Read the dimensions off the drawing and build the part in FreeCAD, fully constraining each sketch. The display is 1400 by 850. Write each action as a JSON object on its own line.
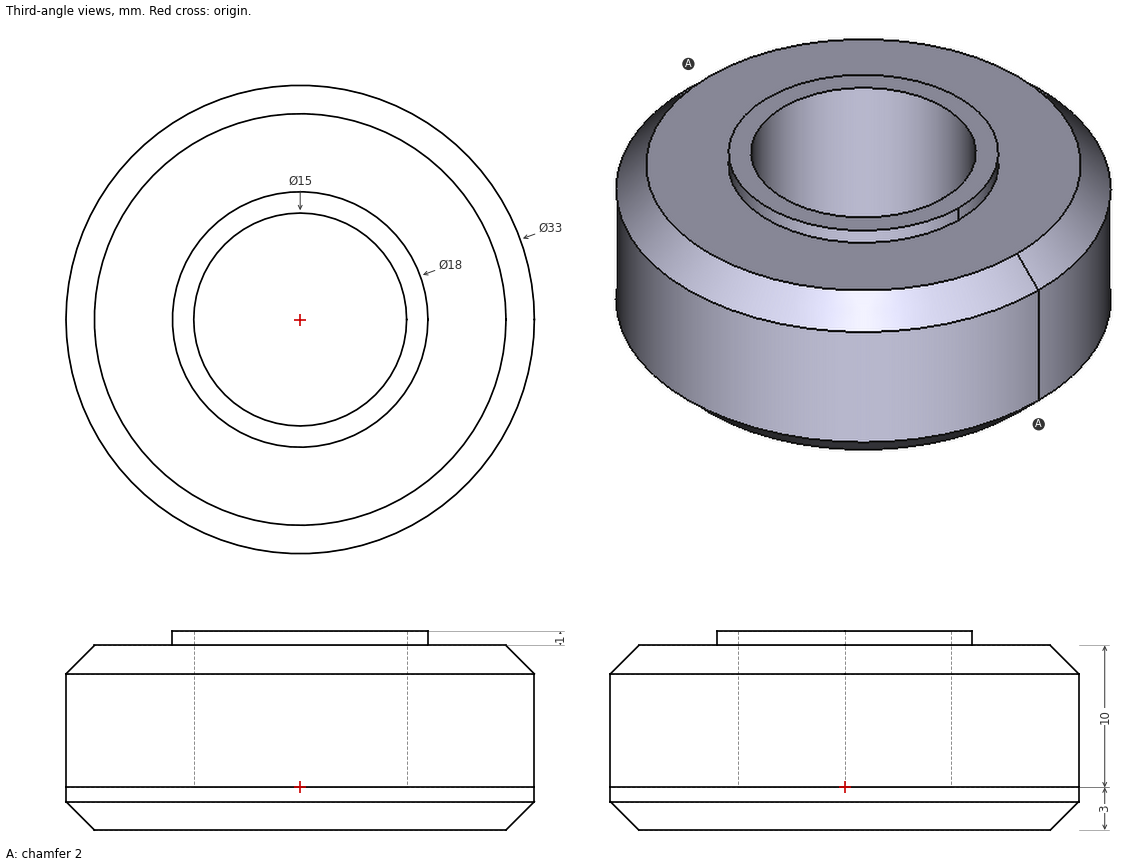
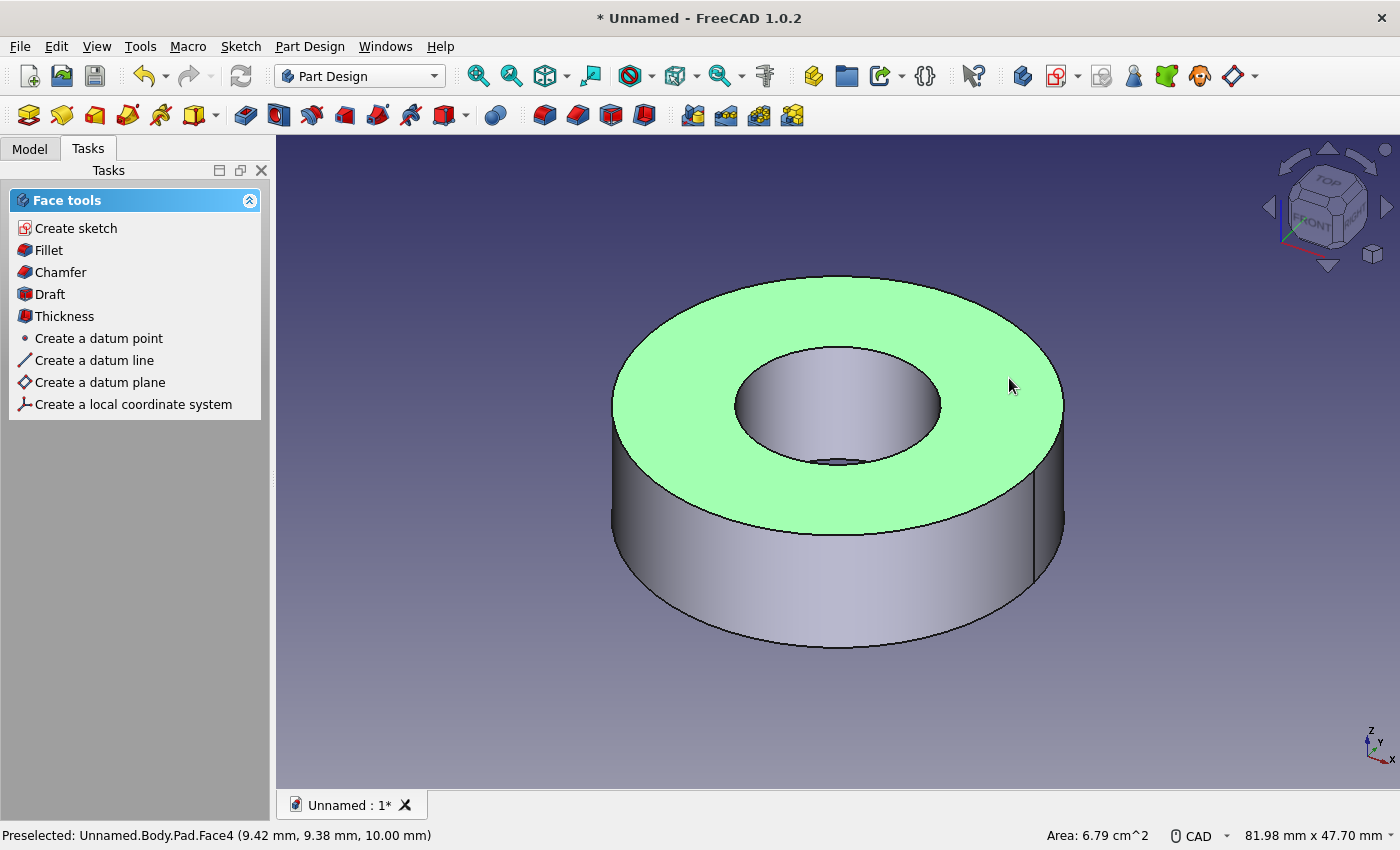
{"action": "left_click", "coordinate": [1056, 76]}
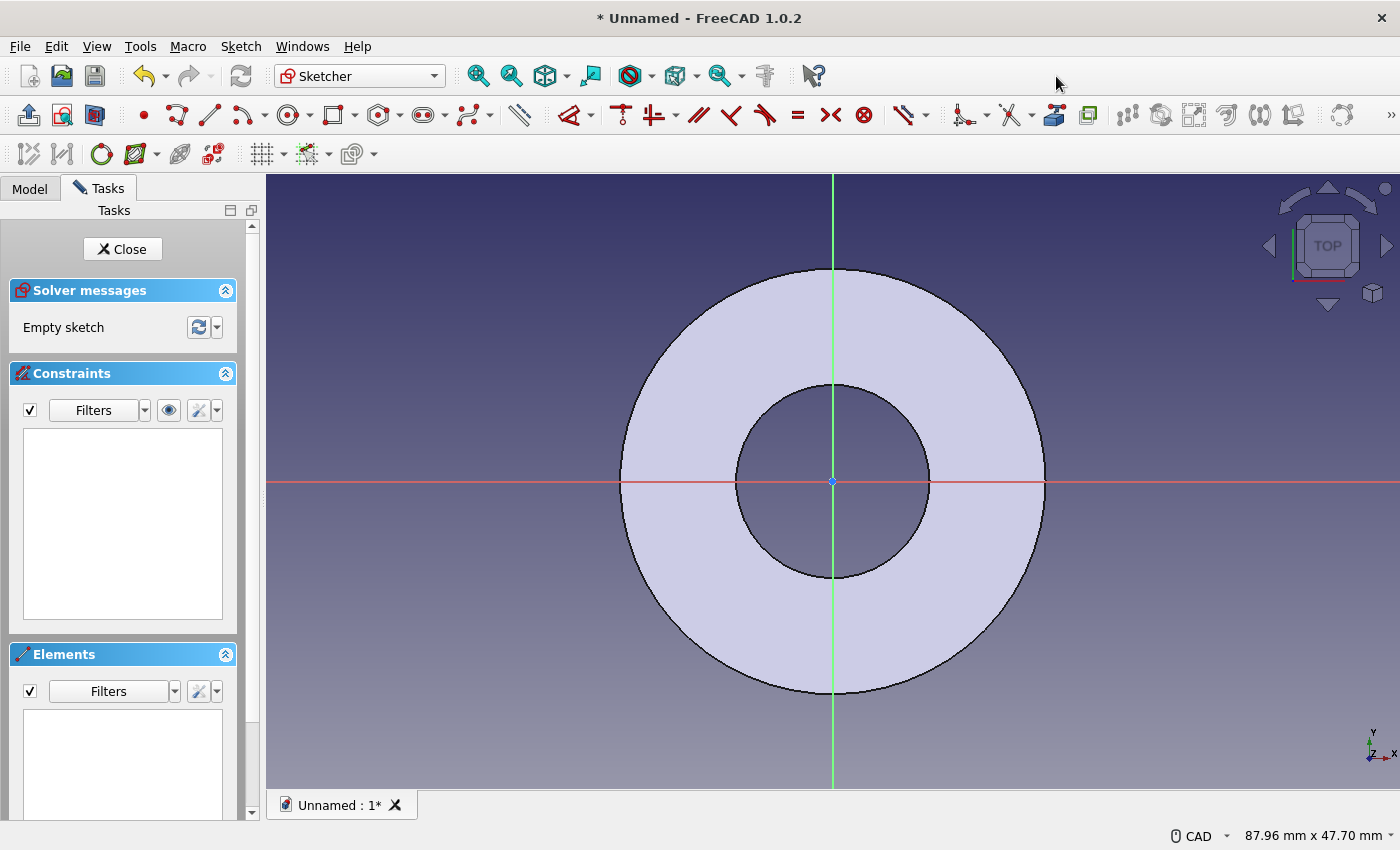
{"action": "scroll", "coordinate": [916, 481], "scroll_direction": "up", "scroll_amount": 3}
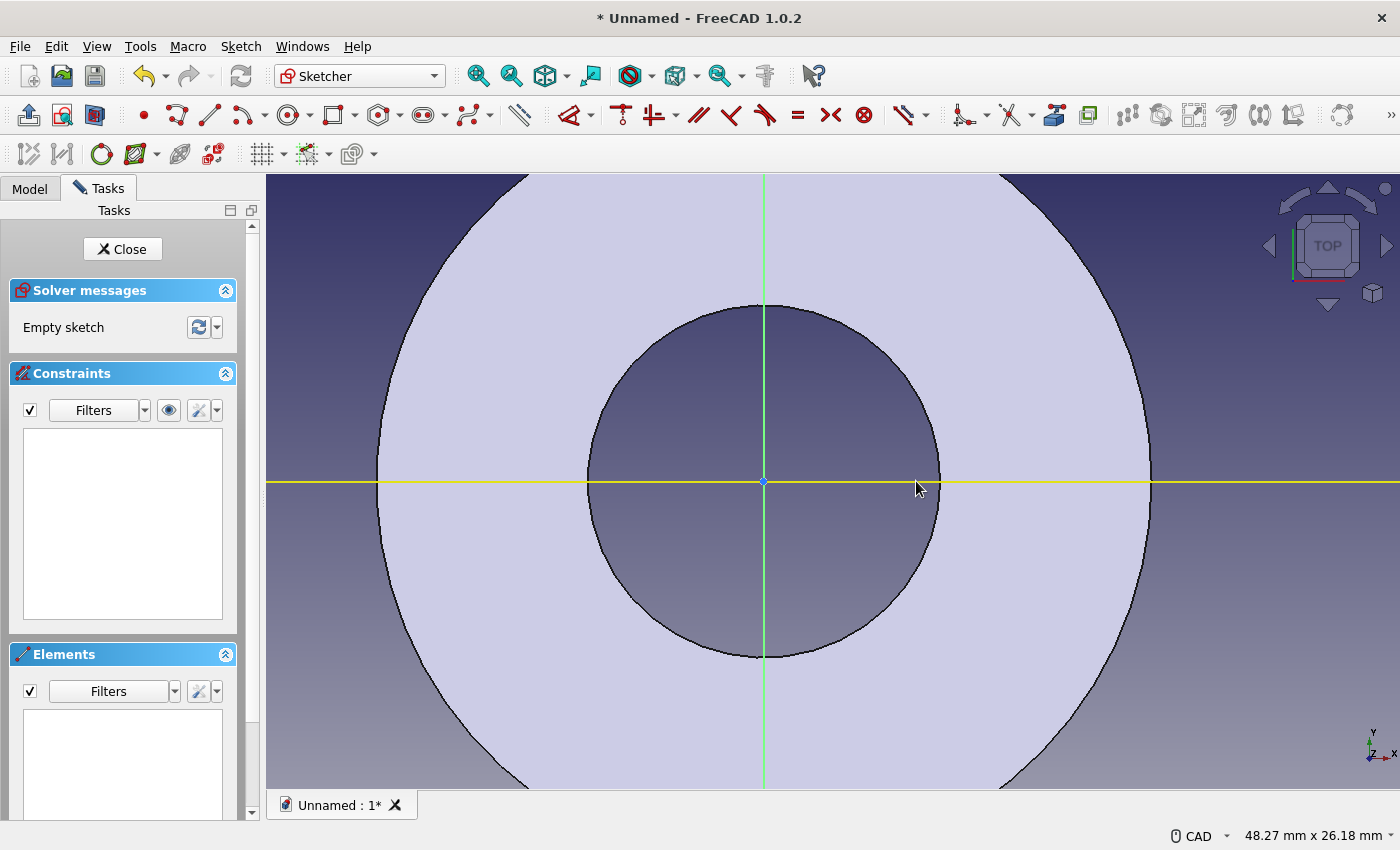
{"action": "key", "text": "g c"}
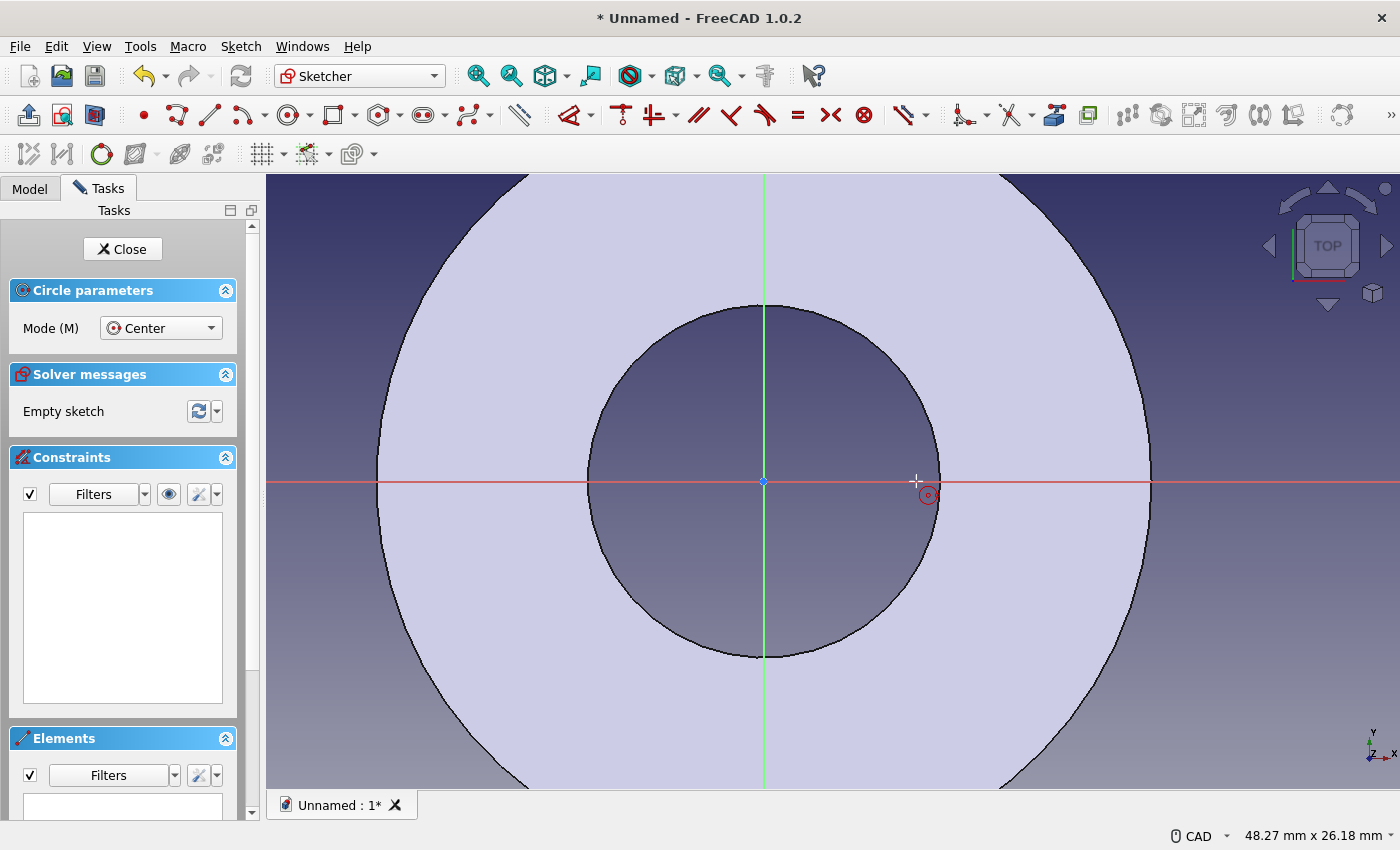
{"action": "left_click", "coordinate": [764, 482]}
{"action": "mouse_move", "coordinate": [913, 332]}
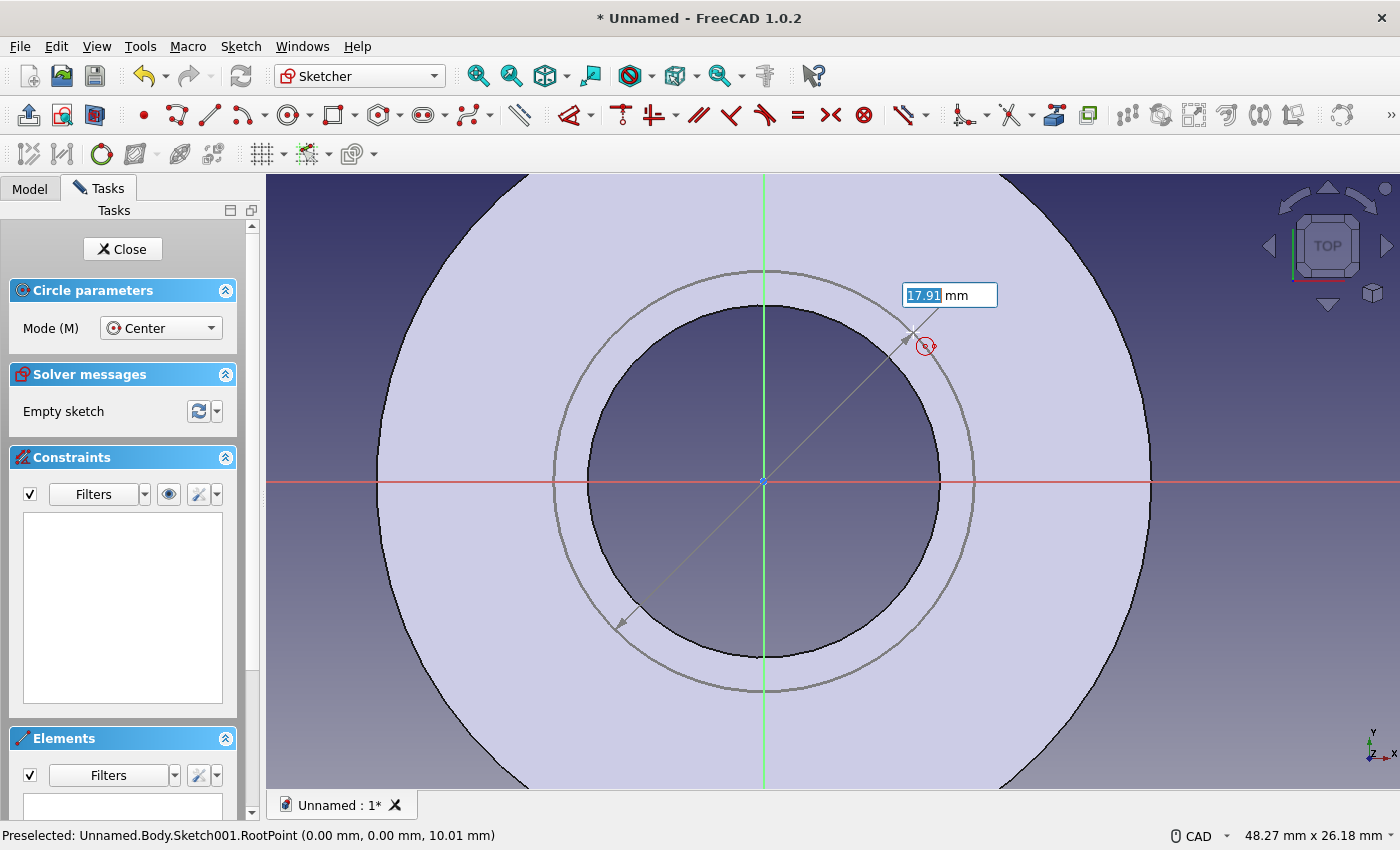
{"action": "type", "text": "18"}
{"action": "key", "text": "Return"}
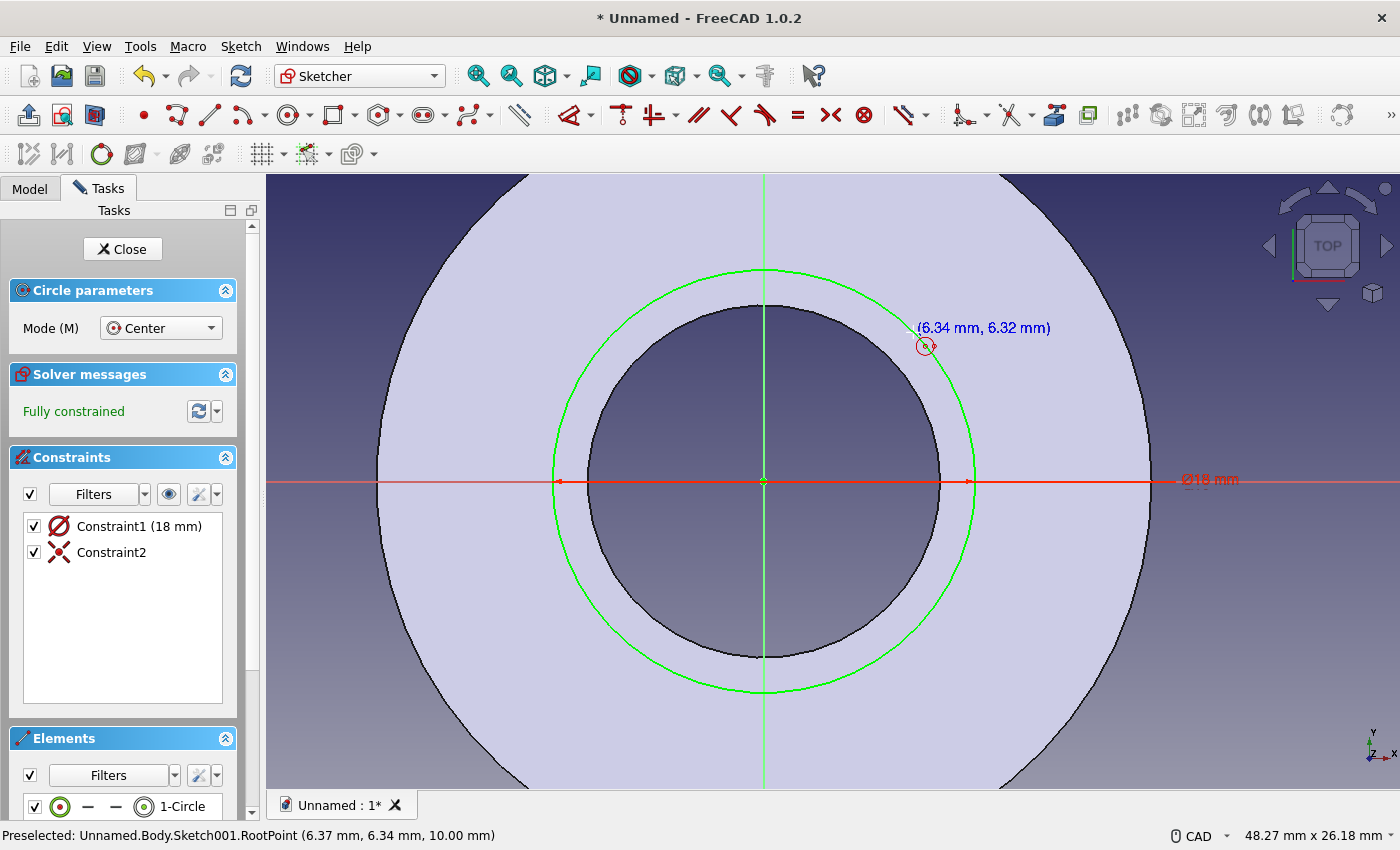
{"action": "left_click", "coordinate": [764, 482]}
{"action": "mouse_move", "coordinate": [889, 357]}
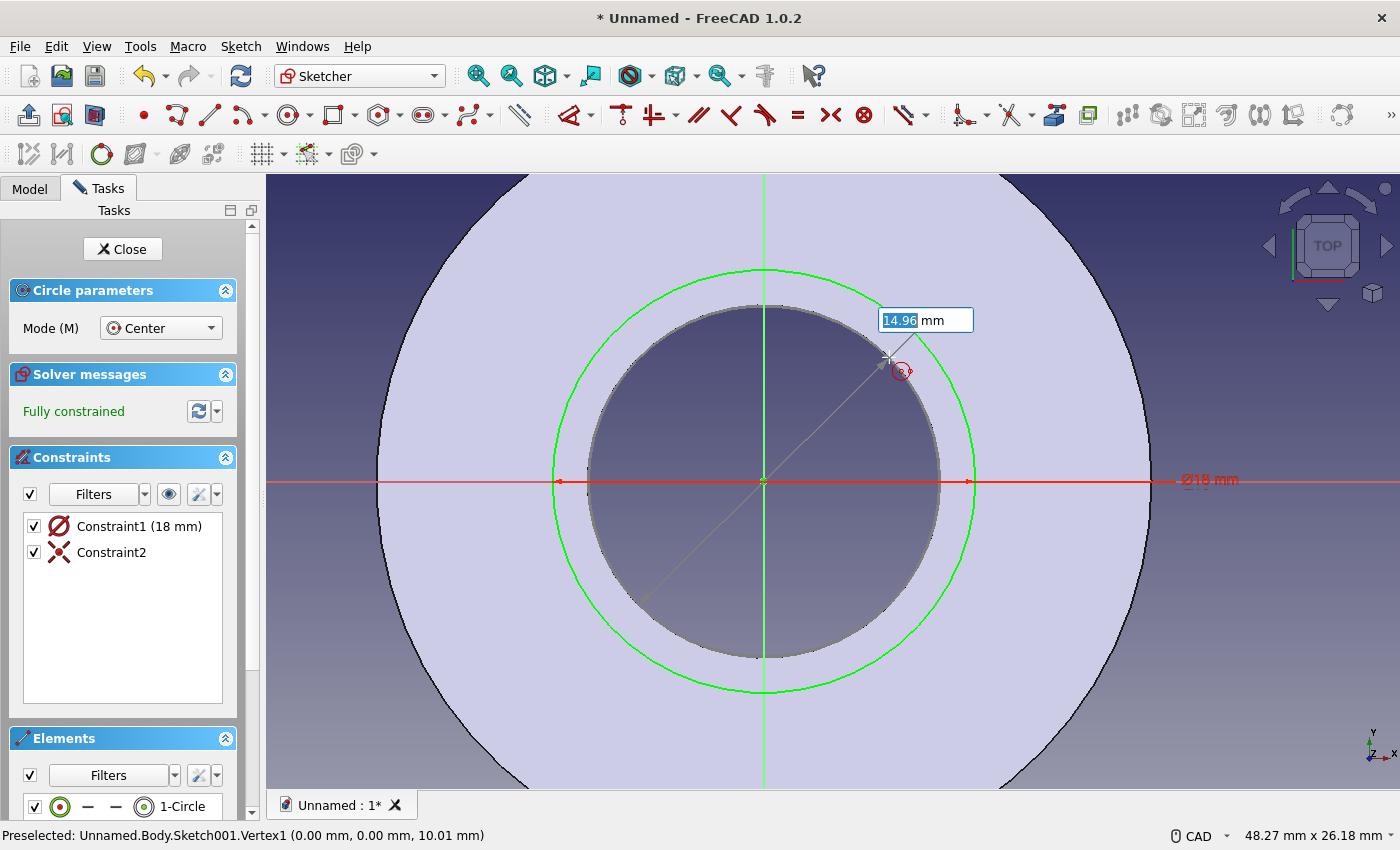
{"action": "type", "text": "15"}
{"action": "key", "text": "Return"}
{"action": "key", "text": "Escape"}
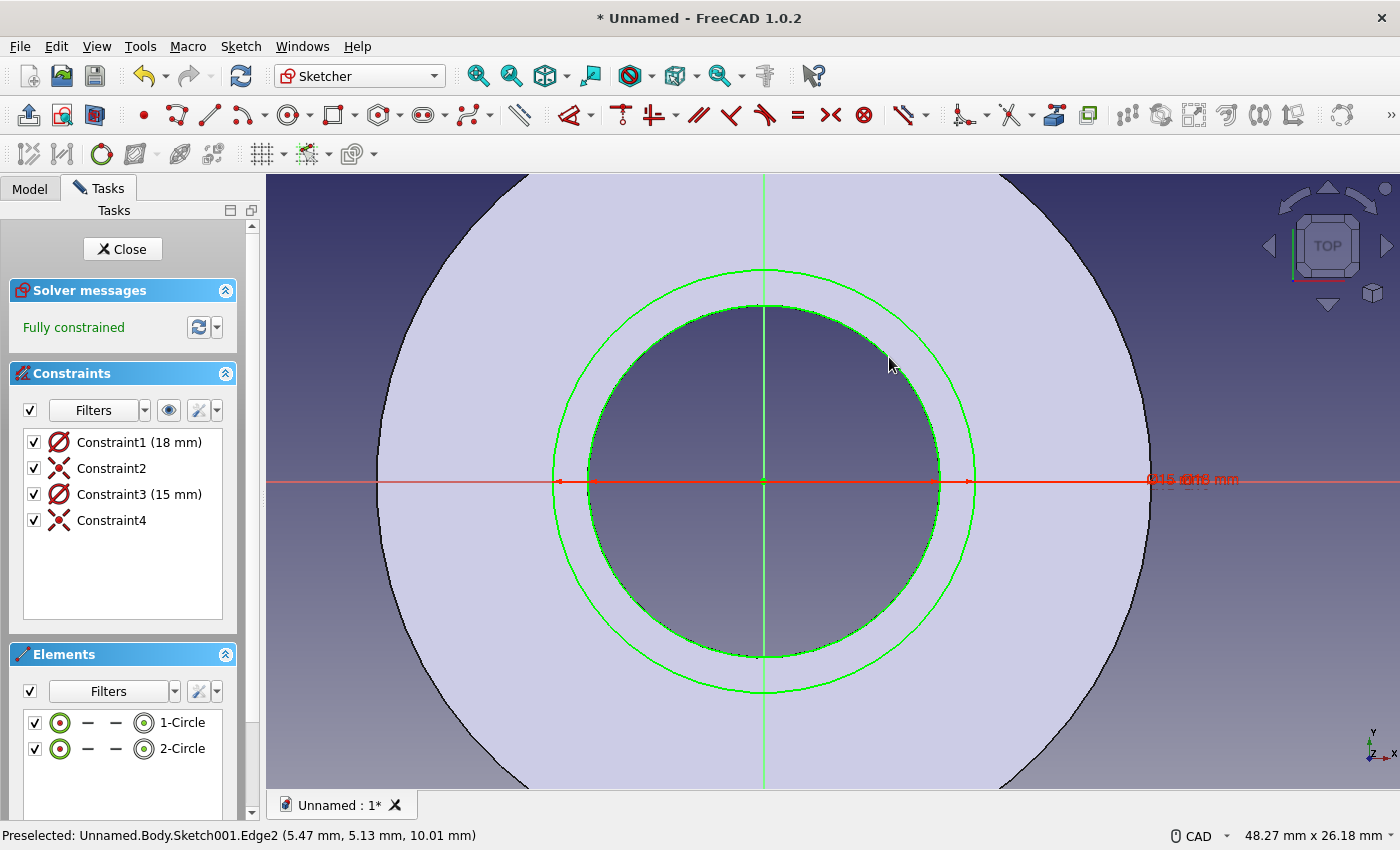
{"action": "left_click", "coordinate": [123, 249]}